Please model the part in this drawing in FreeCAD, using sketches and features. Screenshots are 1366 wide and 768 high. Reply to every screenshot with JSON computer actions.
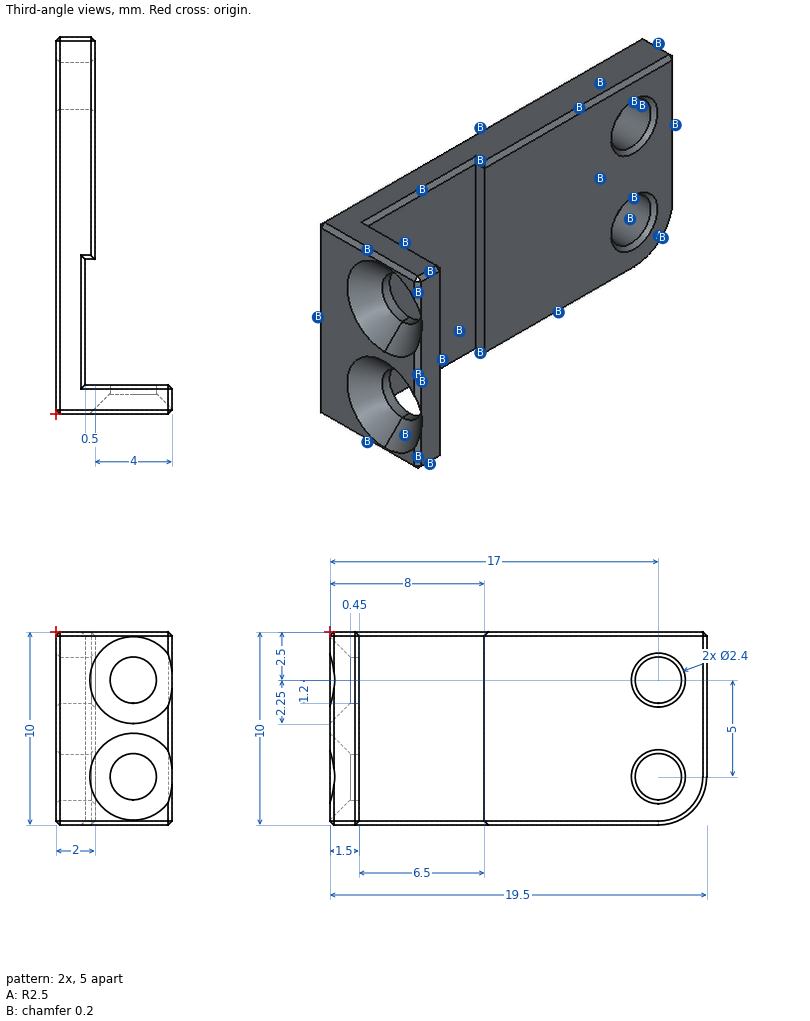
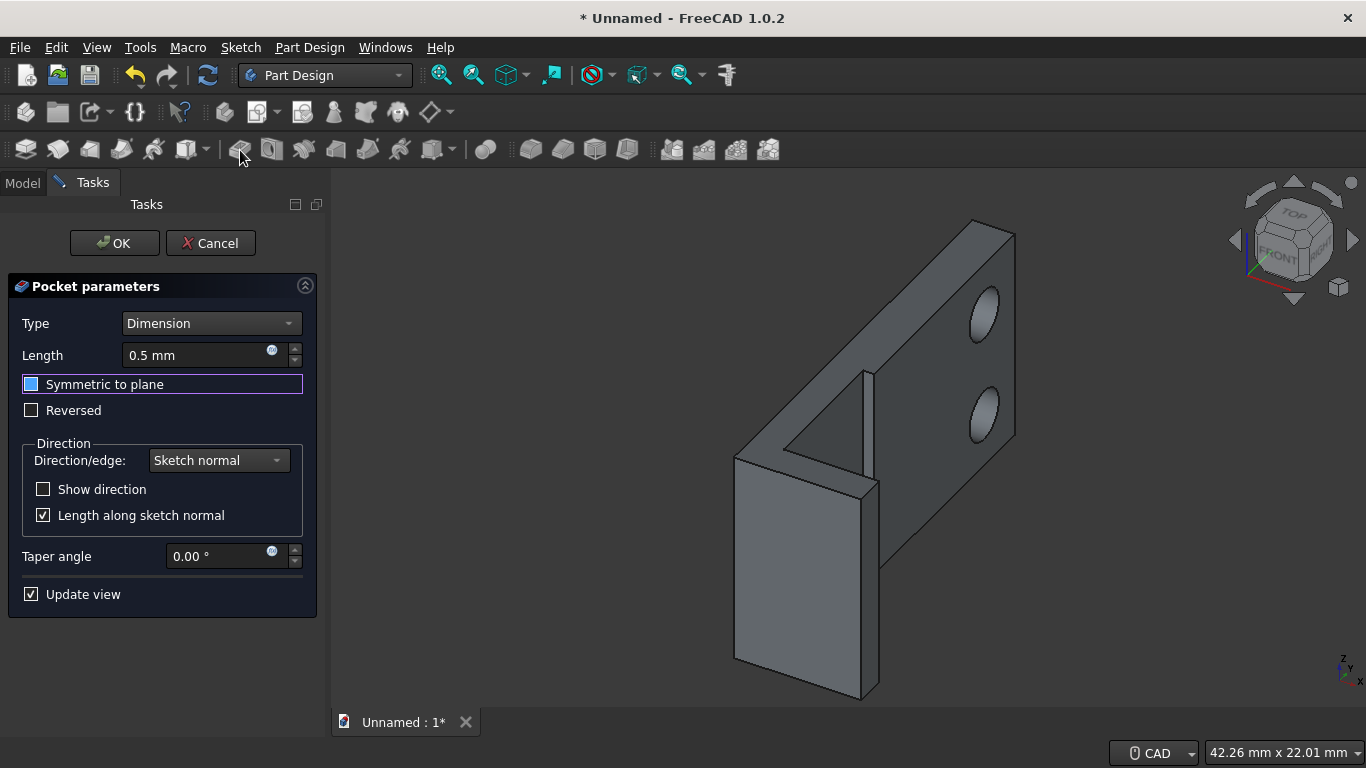
{"action": "left_click", "coordinate": [115, 243]}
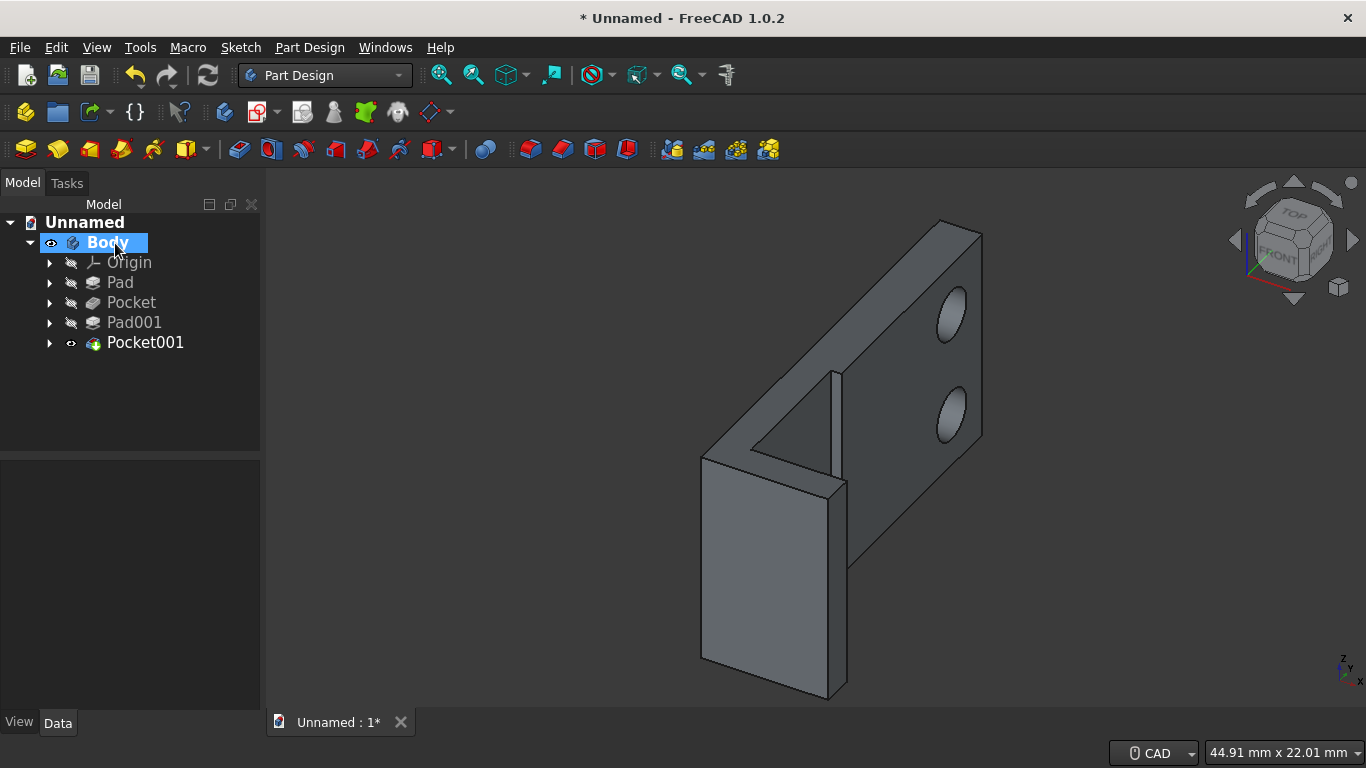
{"action": "left_click", "coordinate": [50, 263]}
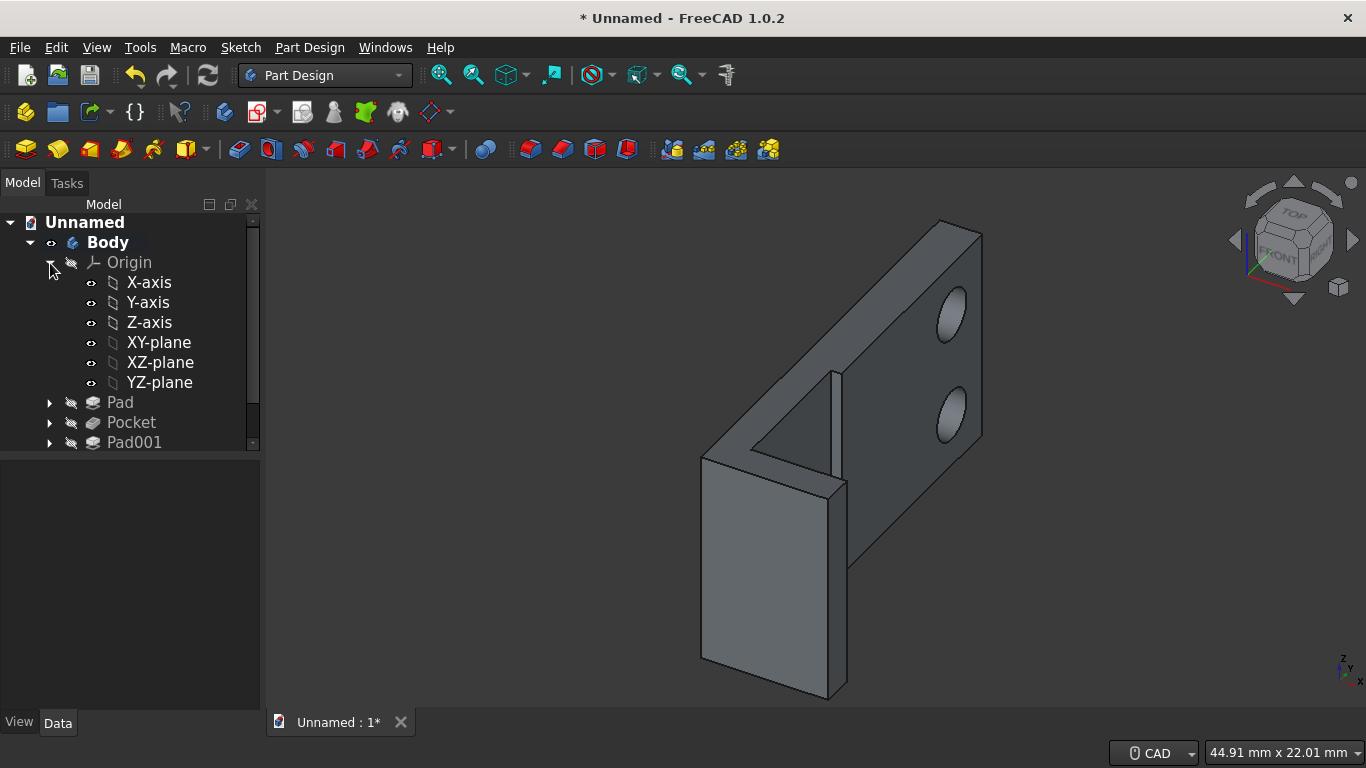
{"action": "left_click", "coordinate": [136, 383]}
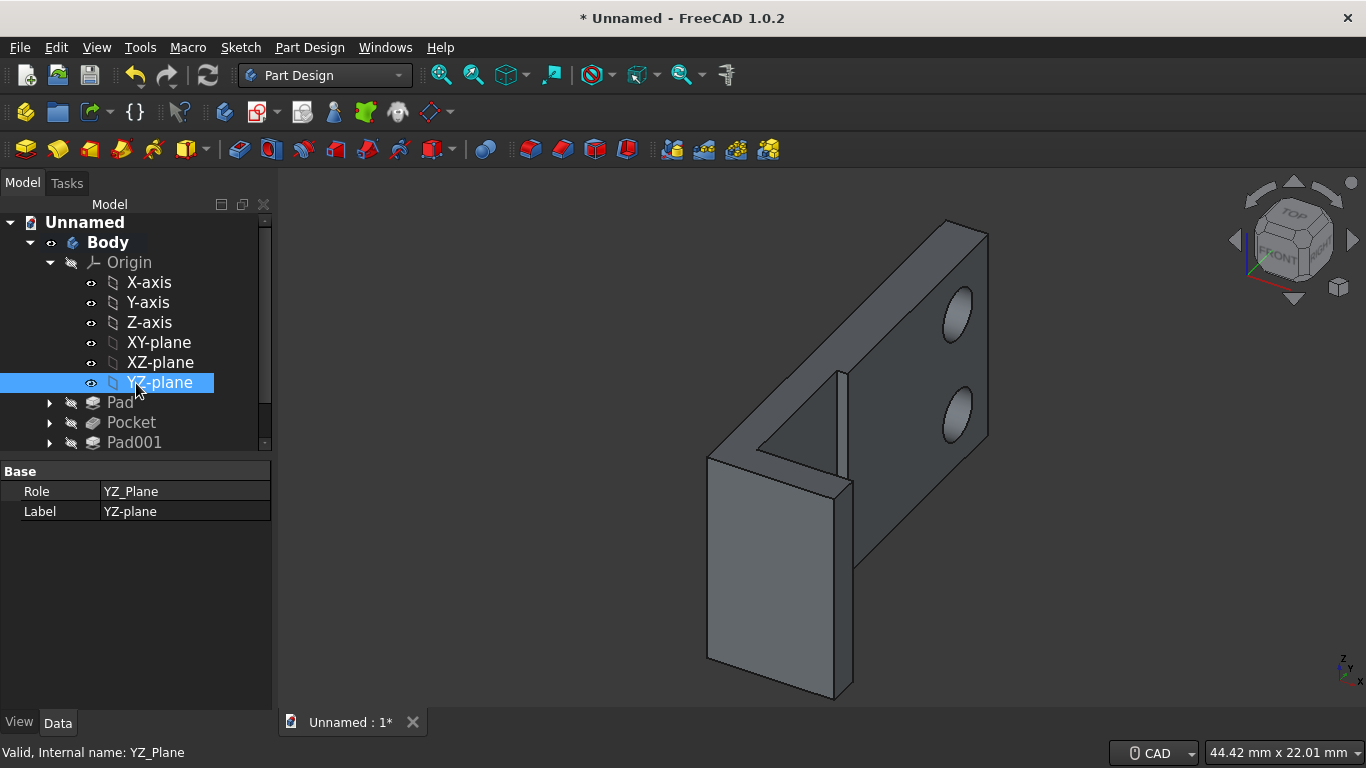
{"action": "left_click", "coordinate": [430, 112]}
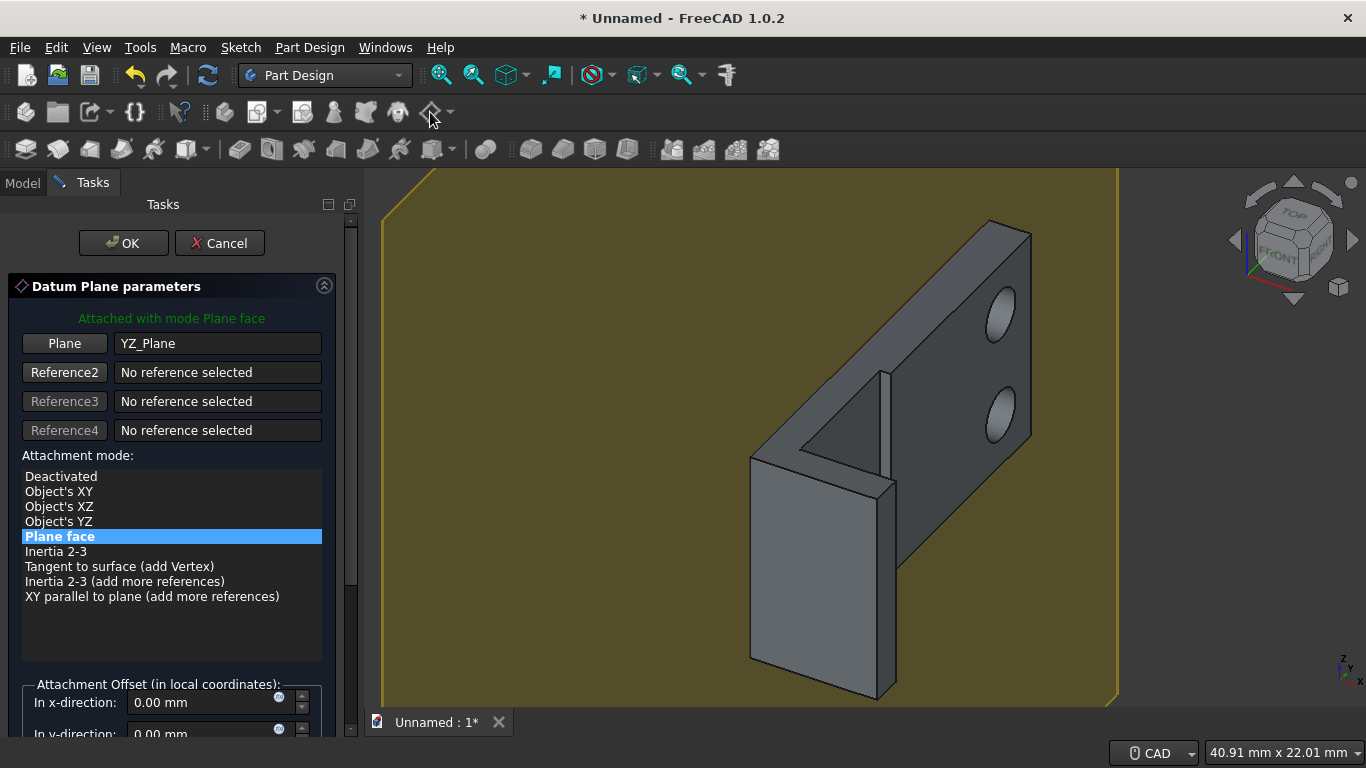
{"action": "scroll", "coordinate": [351, 475], "scroll_direction": "down", "scroll_amount": 2}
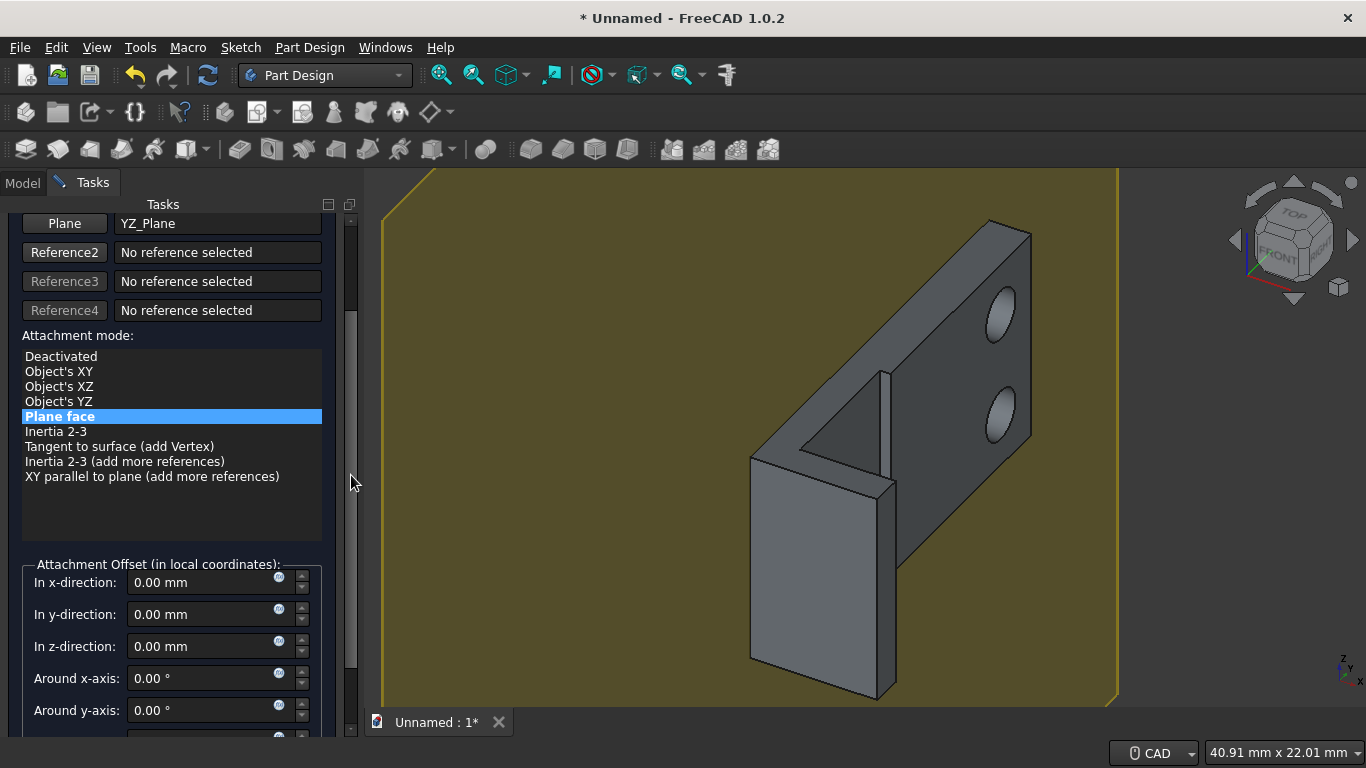
{"action": "triple_click", "coordinate": [210, 646]}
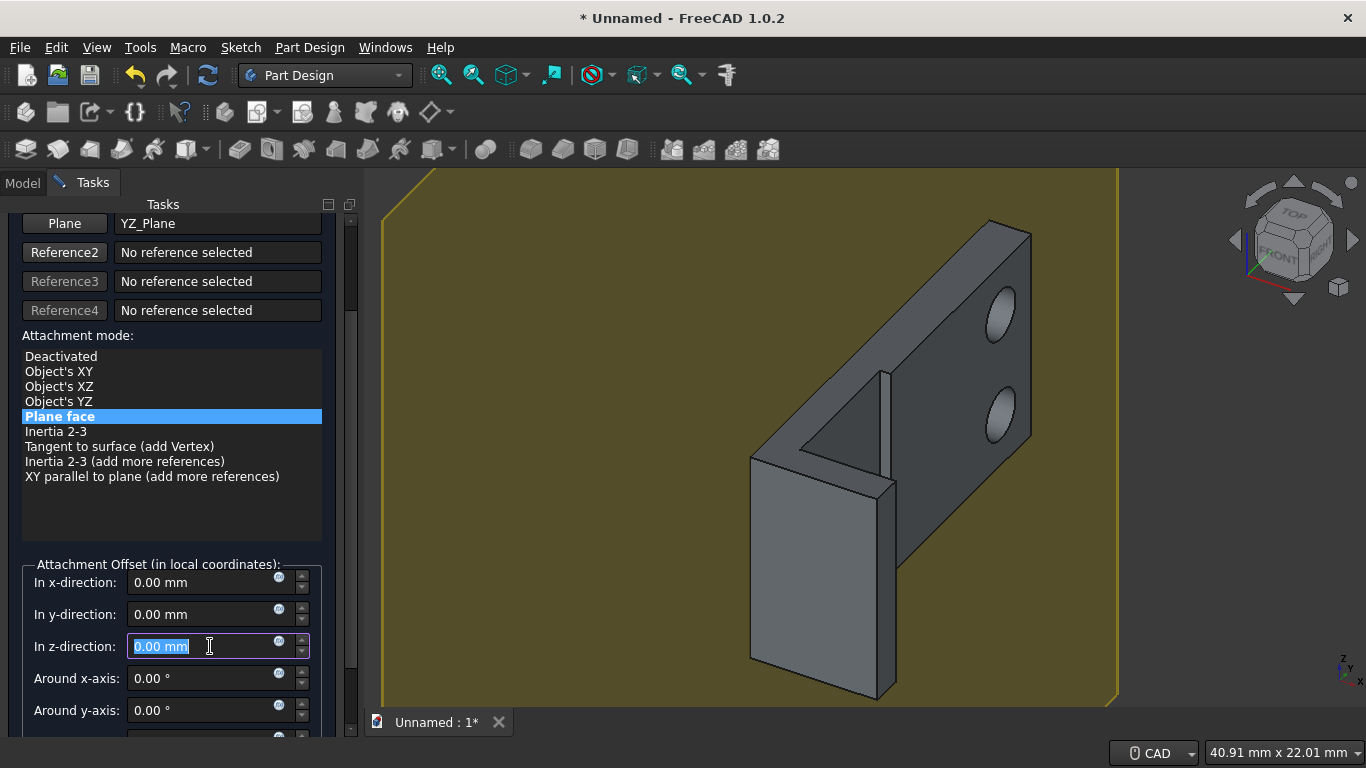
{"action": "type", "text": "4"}
{"action": "key", "text": "Tab"}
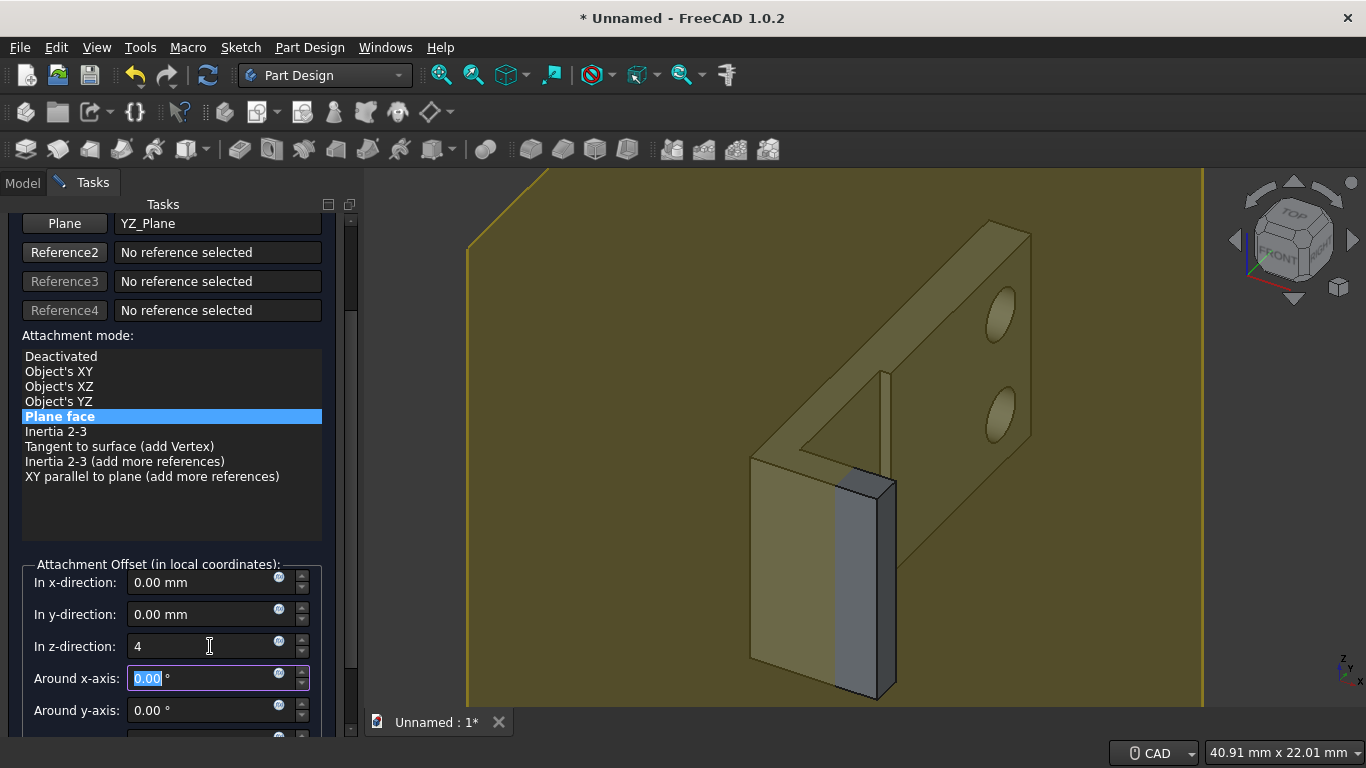
{"action": "scroll", "coordinate": [351, 475], "scroll_direction": "up", "scroll_amount": 3}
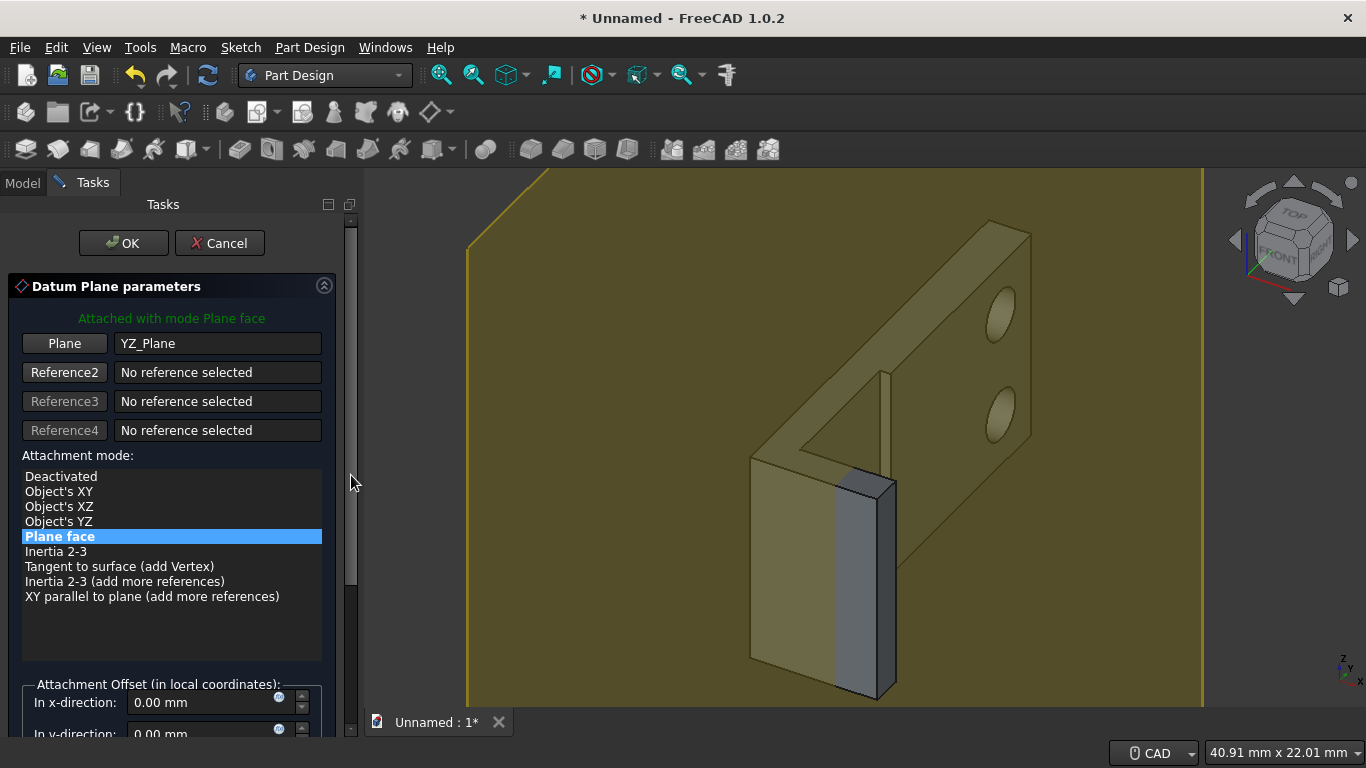
{"action": "left_click", "coordinate": [124, 243]}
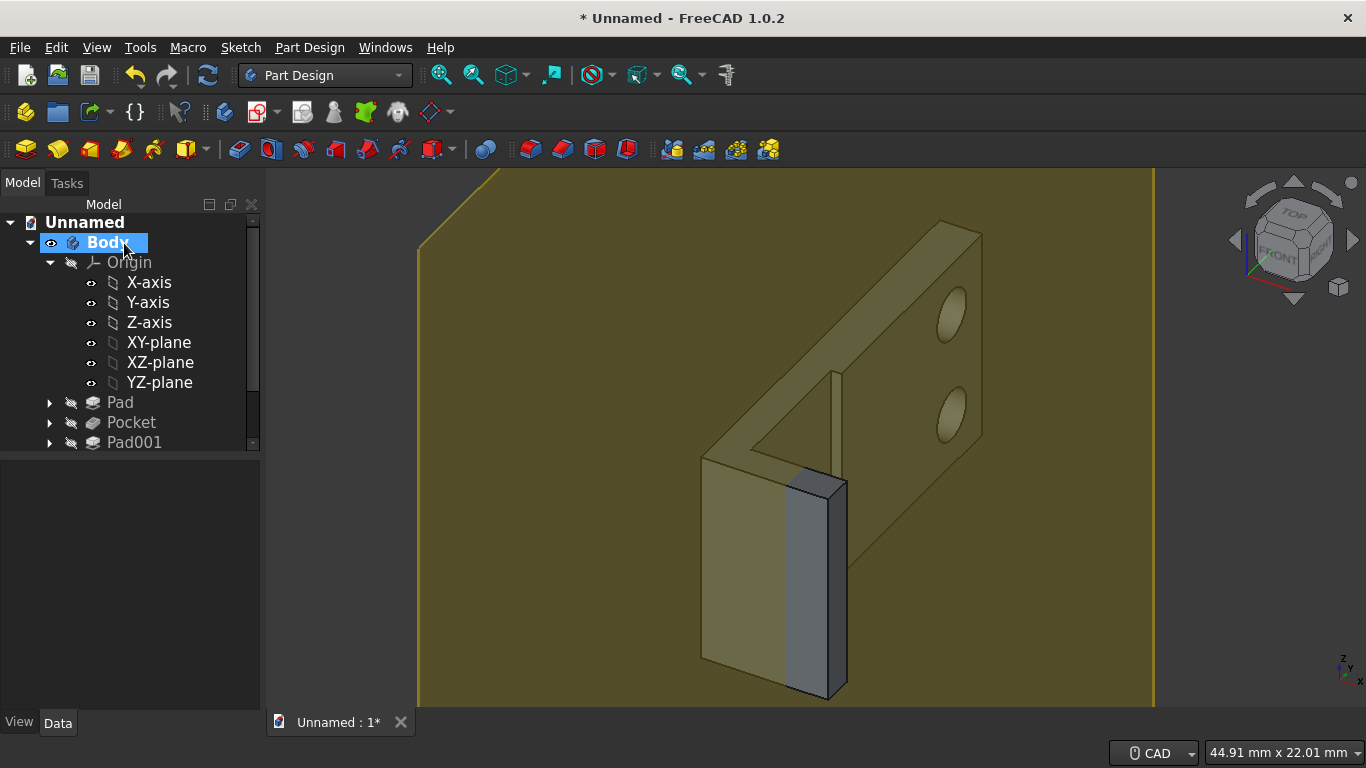
{"action": "scroll", "coordinate": [100, 338], "scroll_direction": "down", "scroll_amount": 3}